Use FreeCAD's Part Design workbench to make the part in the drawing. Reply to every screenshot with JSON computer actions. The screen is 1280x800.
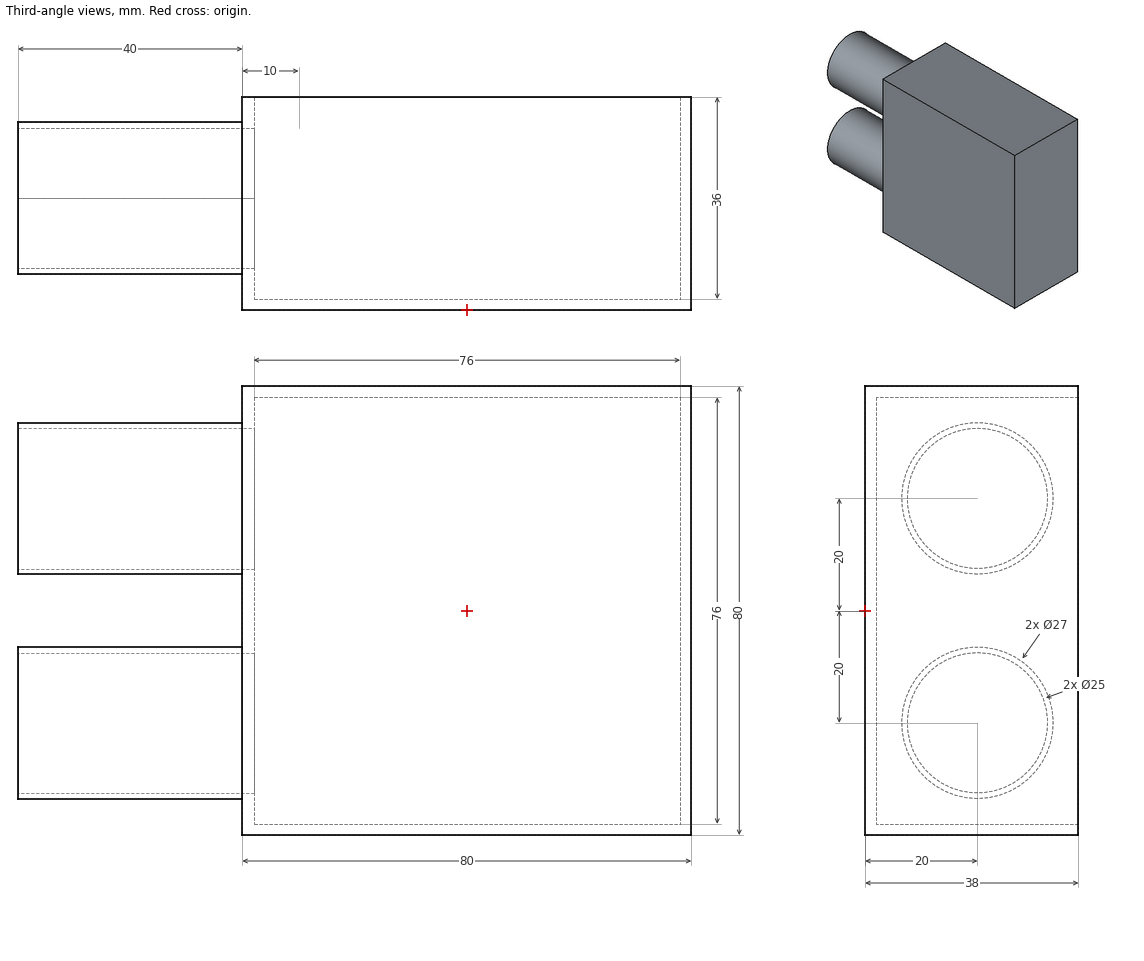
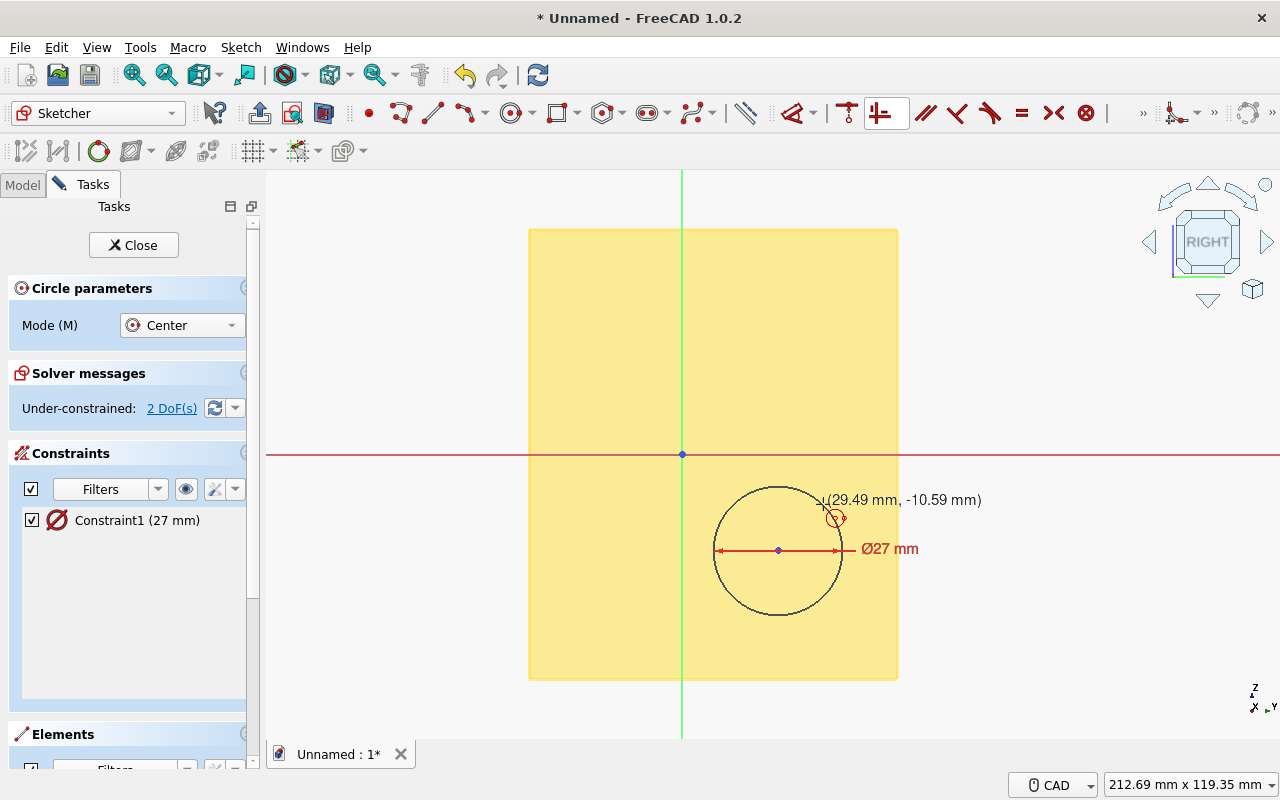
{"action": "left_click", "coordinate": [778, 359]}
{"action": "mouse_move", "coordinate": [823, 314]}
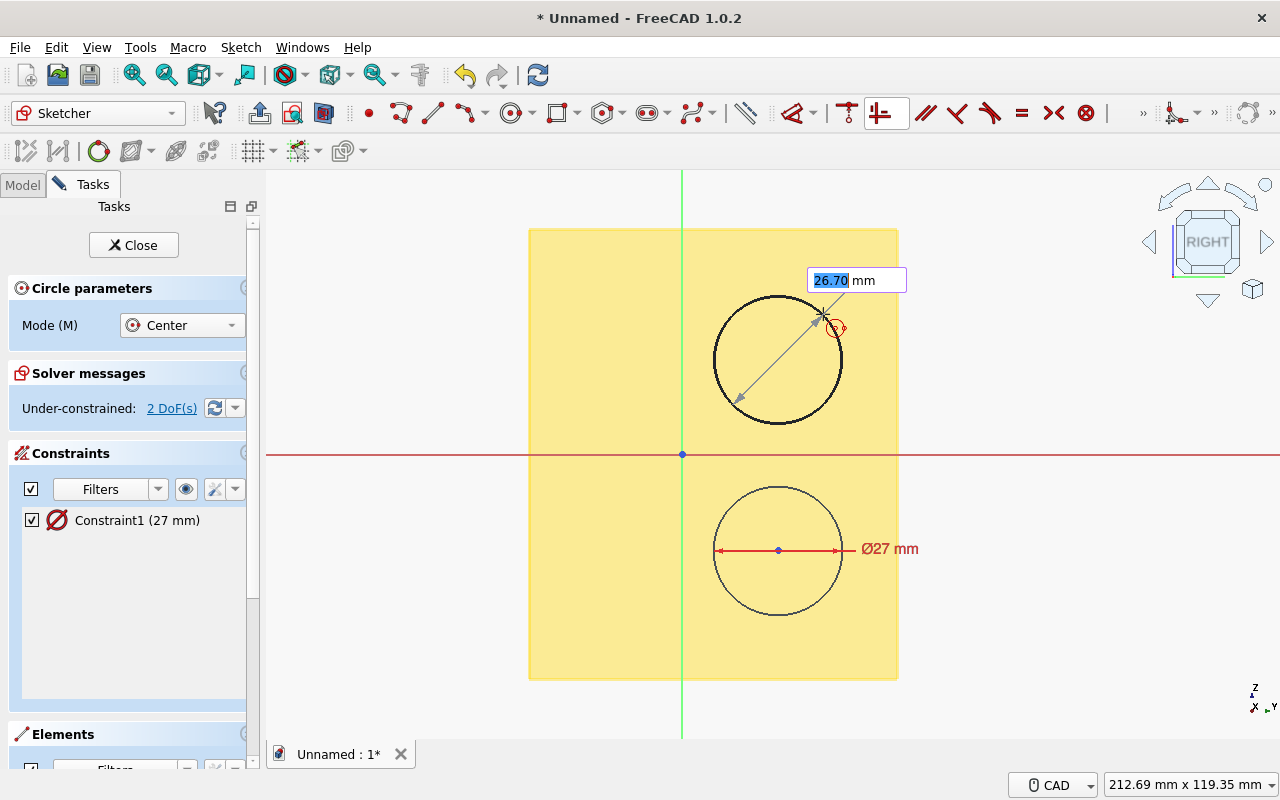
{"action": "type", "text": "27"}
{"action": "key", "text": "Return"}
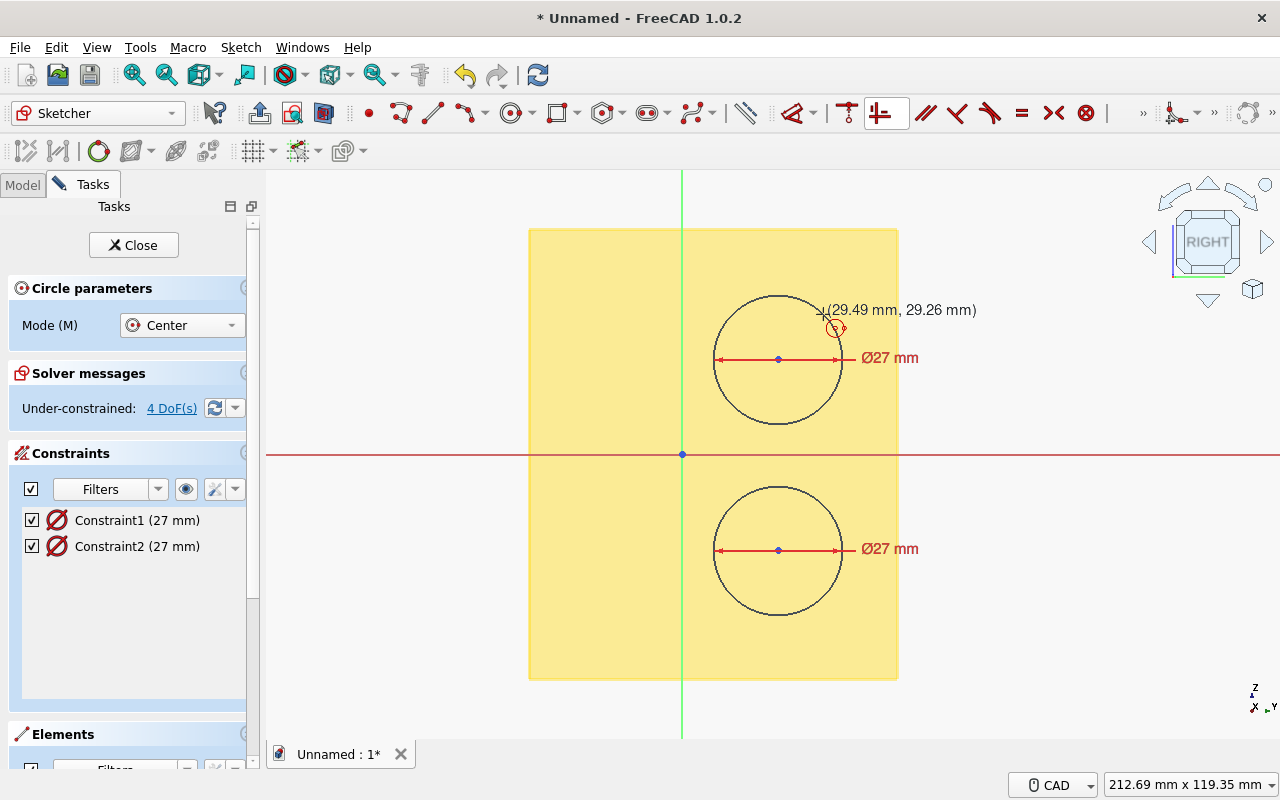
{"action": "left_click", "coordinate": [778, 551]}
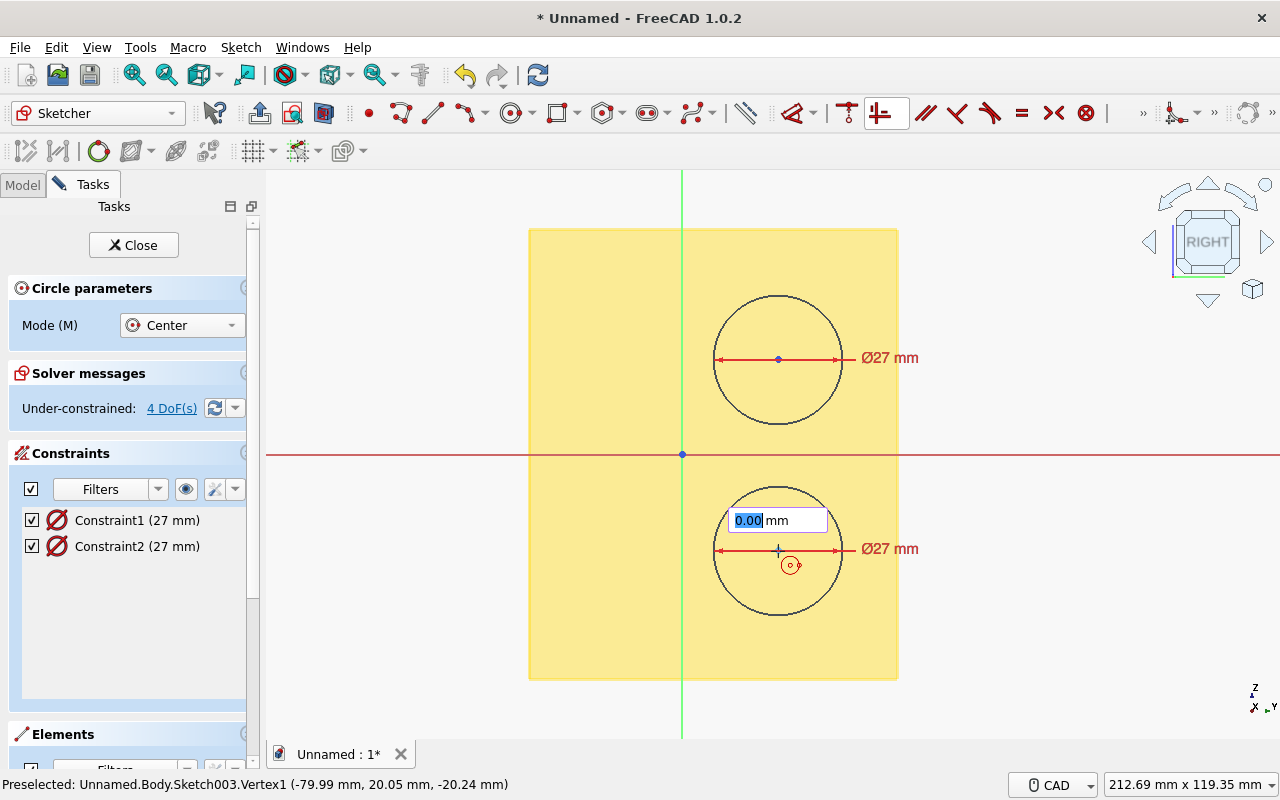
{"action": "scroll", "coordinate": [820, 508], "scroll_direction": "up", "scroll_amount": 7}
{"action": "mouse_move", "coordinate": [818, 505]}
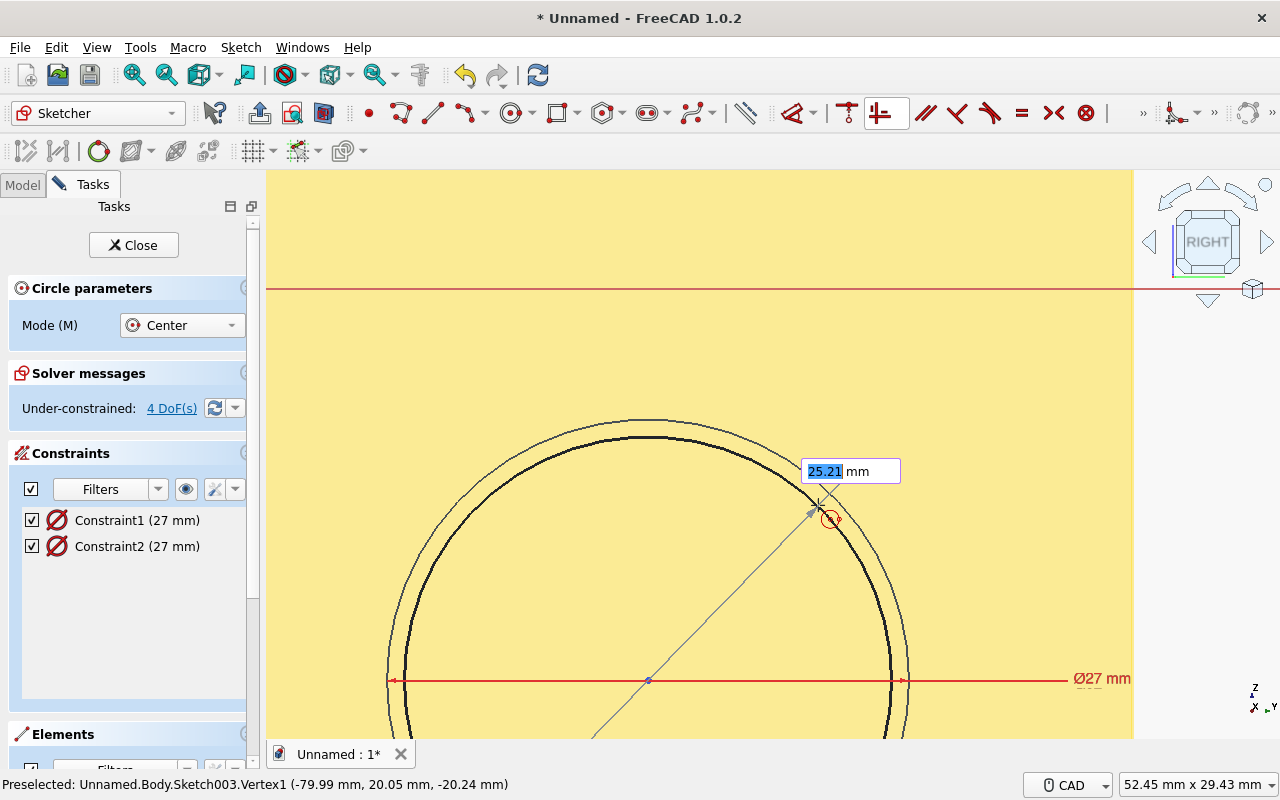
{"action": "type", "text": "25"}
{"action": "key", "text": "Return"}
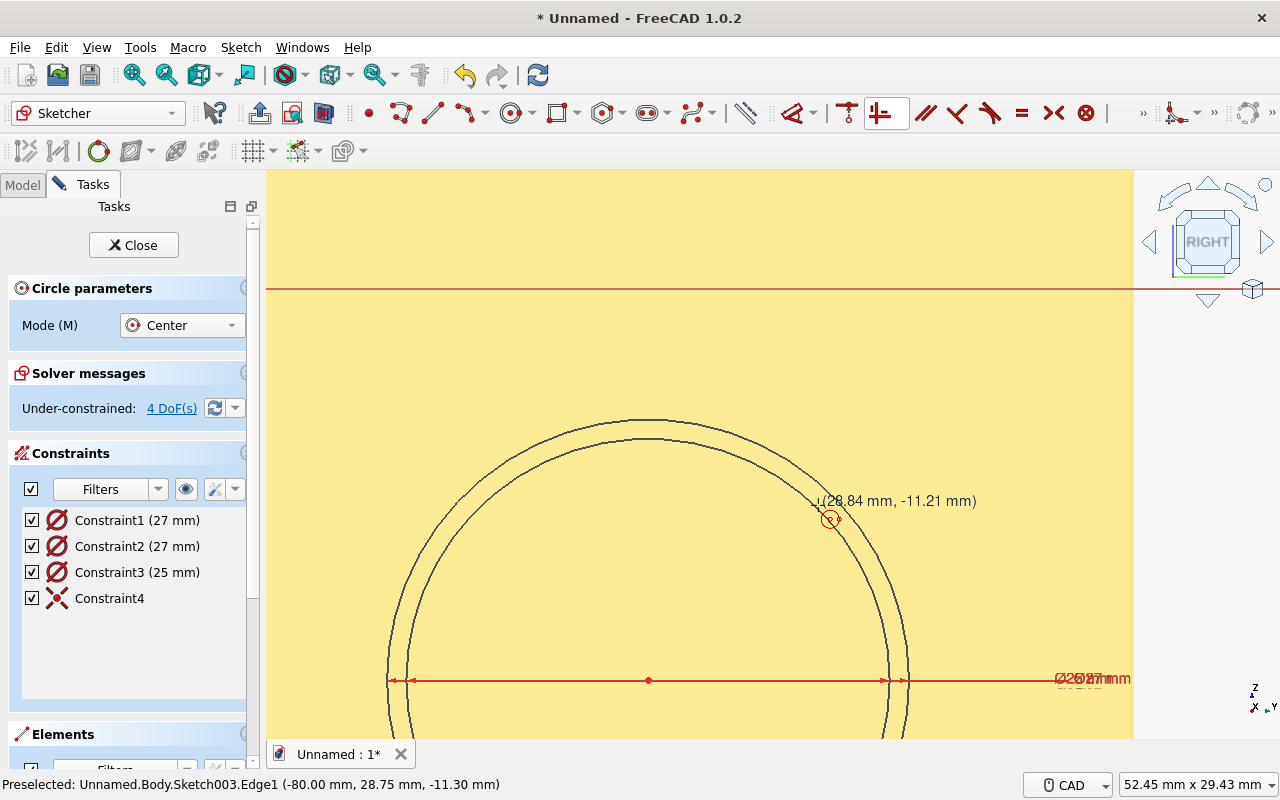
{"action": "scroll", "coordinate": [756, 526], "scroll_direction": "down", "scroll_amount": 6}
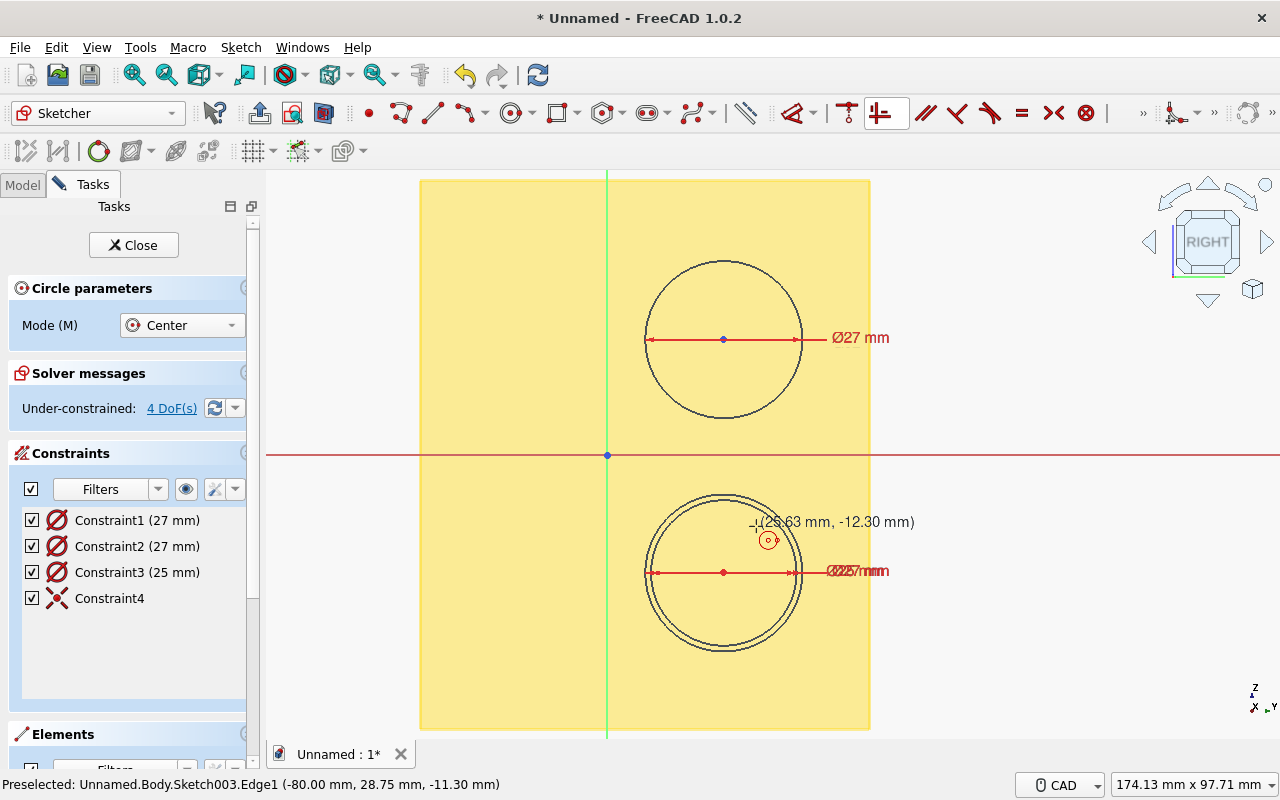
{"action": "left_click", "coordinate": [724, 340]}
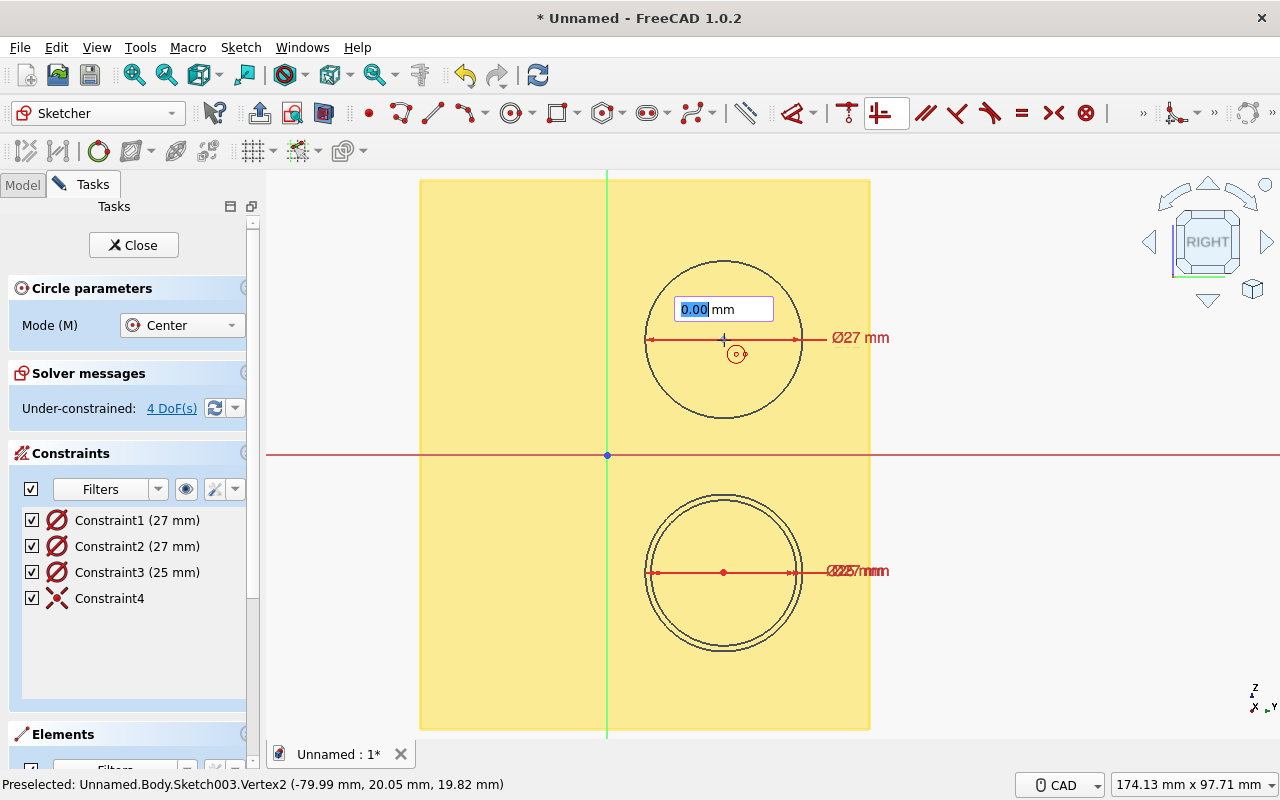
{"action": "scroll", "coordinate": [748, 270], "scroll_direction": "up", "scroll_amount": 6}
{"action": "mouse_move", "coordinate": [748, 270]}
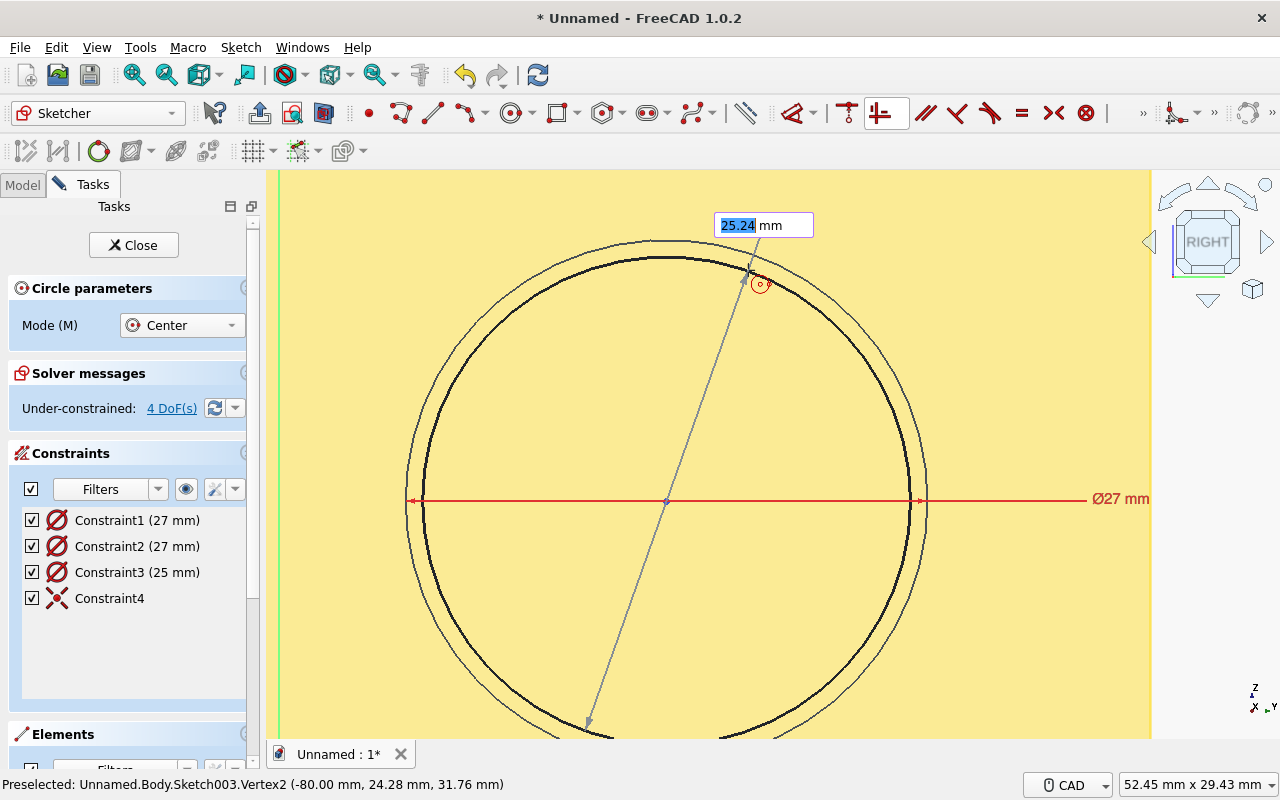
{"action": "type", "text": "25"}
{"action": "key", "text": "Return"}
{"action": "key", "text": "Escape"}